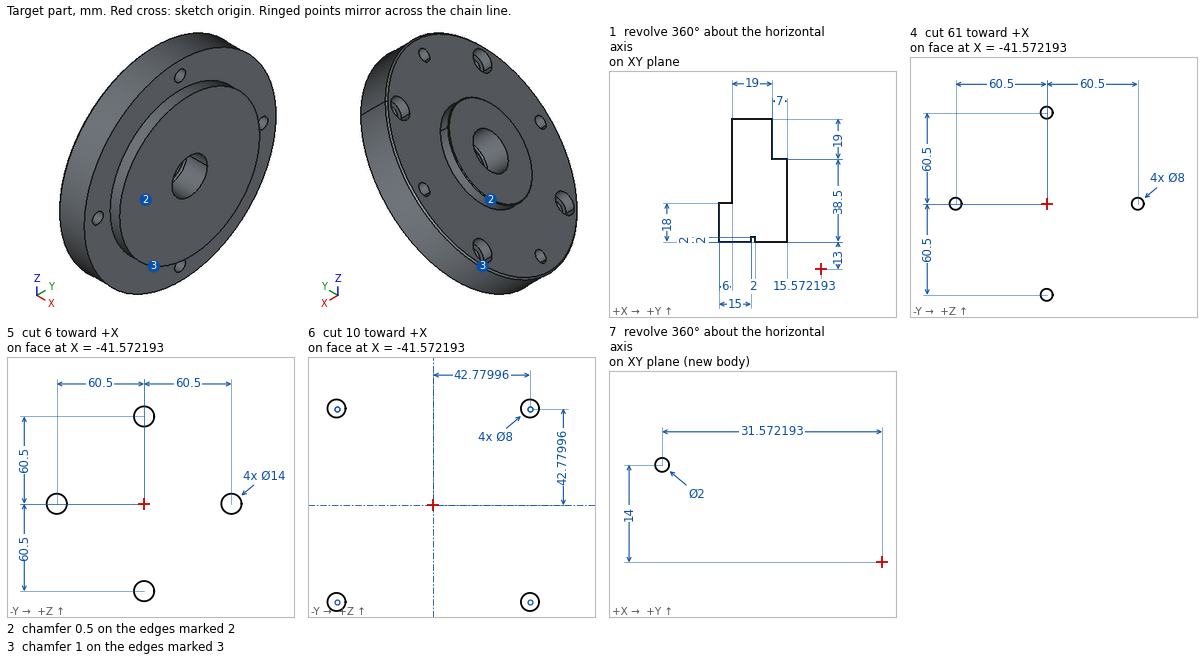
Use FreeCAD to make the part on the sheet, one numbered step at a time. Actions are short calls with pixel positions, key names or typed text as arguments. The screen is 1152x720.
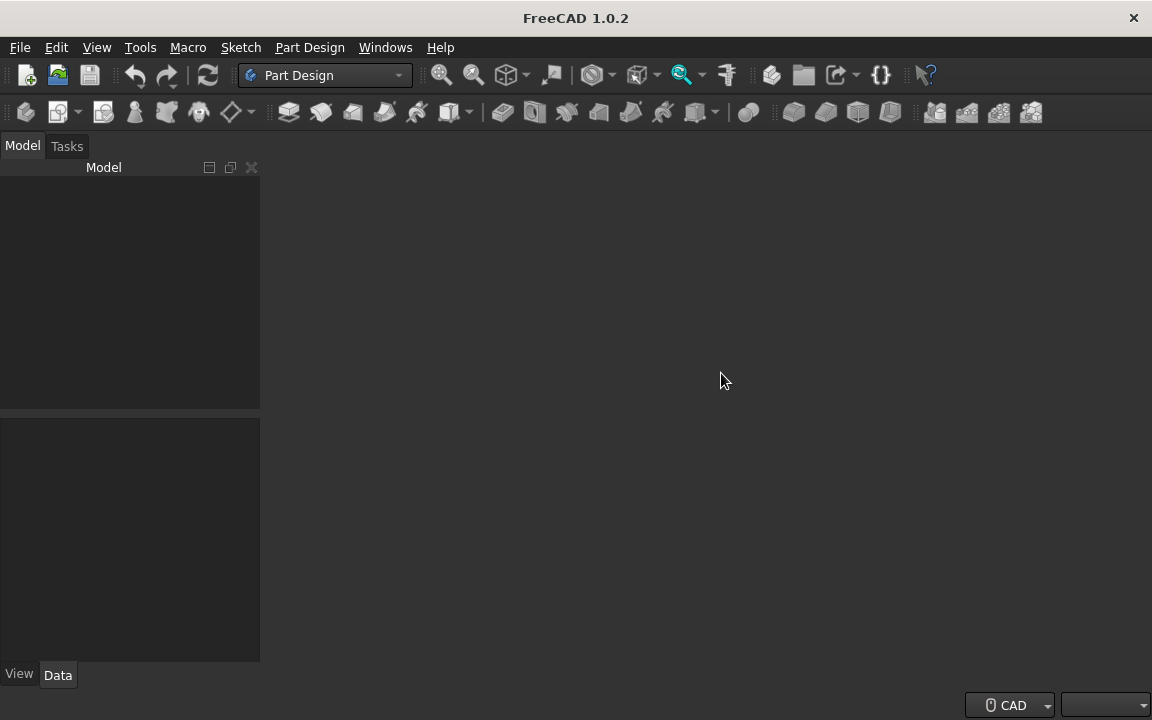
click(26, 76)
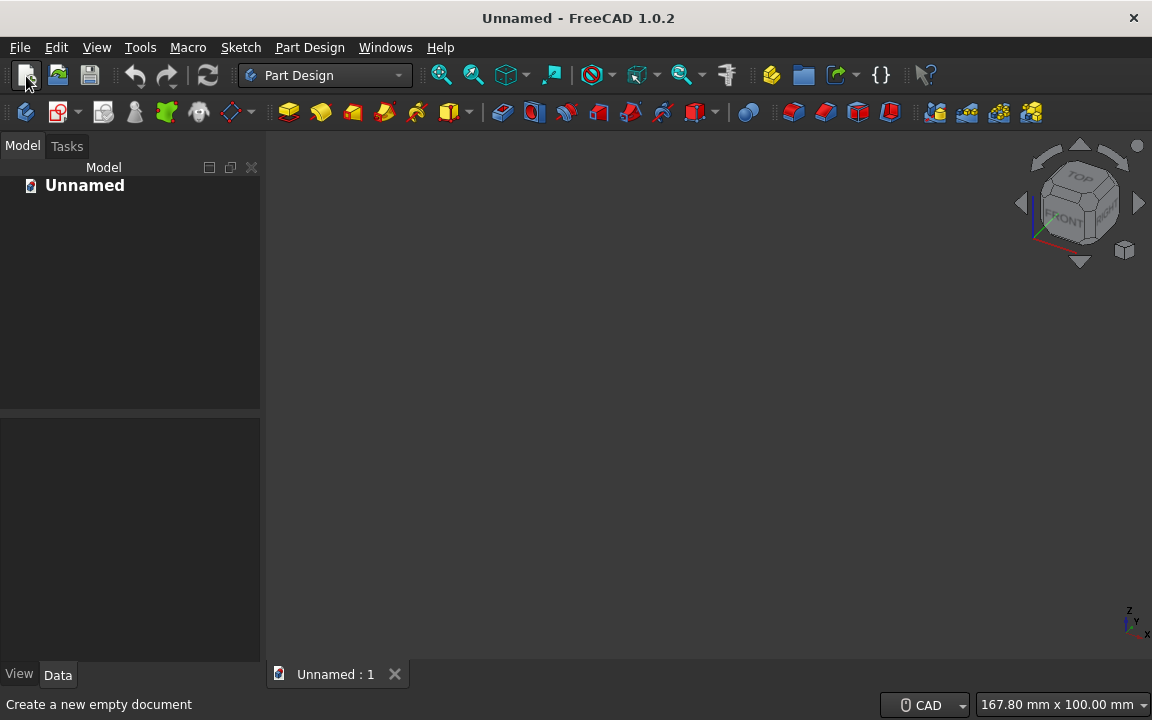
click(58, 112)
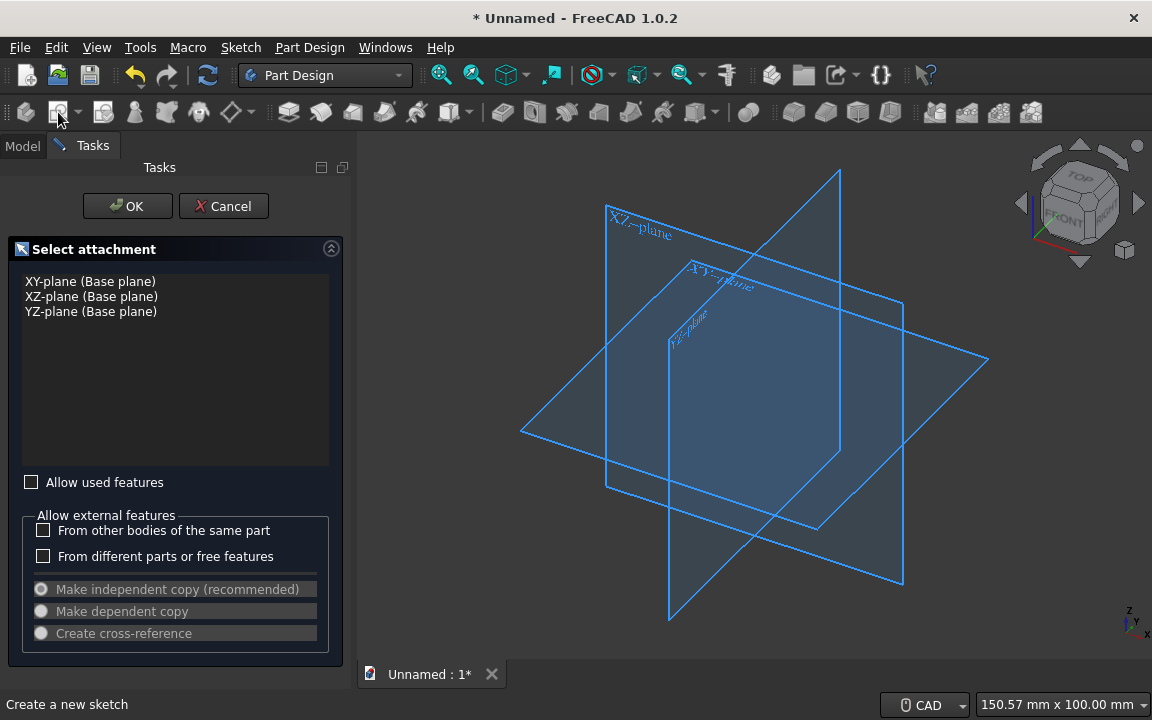
click(82, 282)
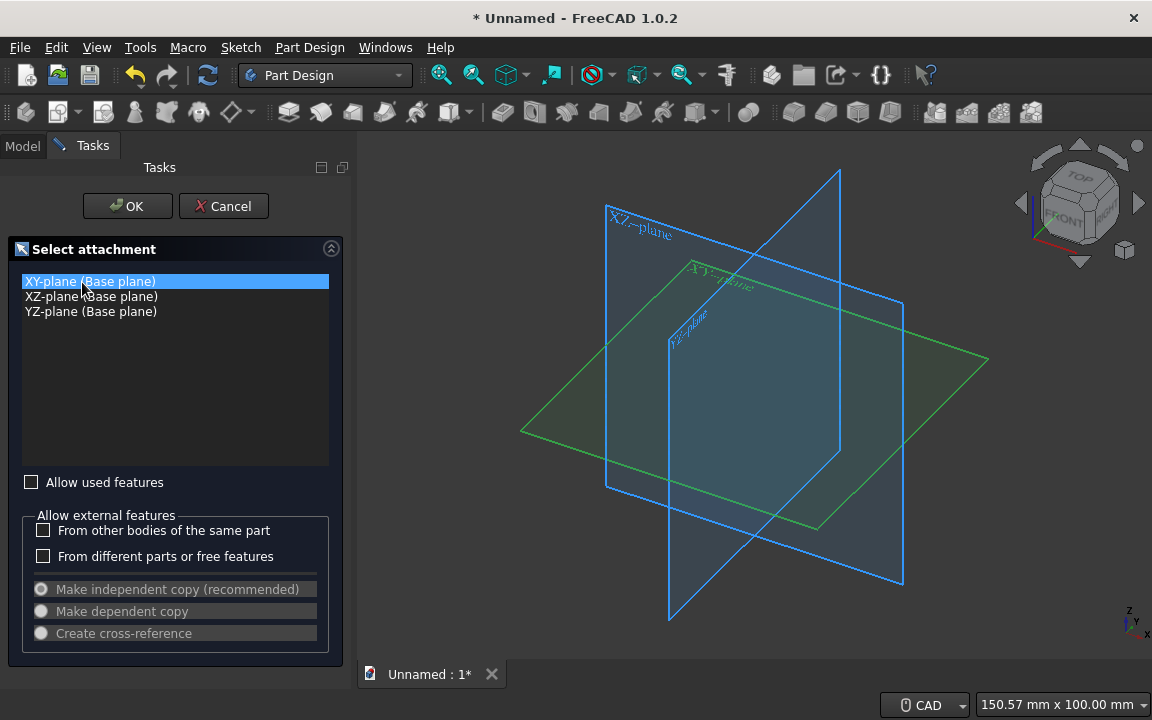
click(128, 206)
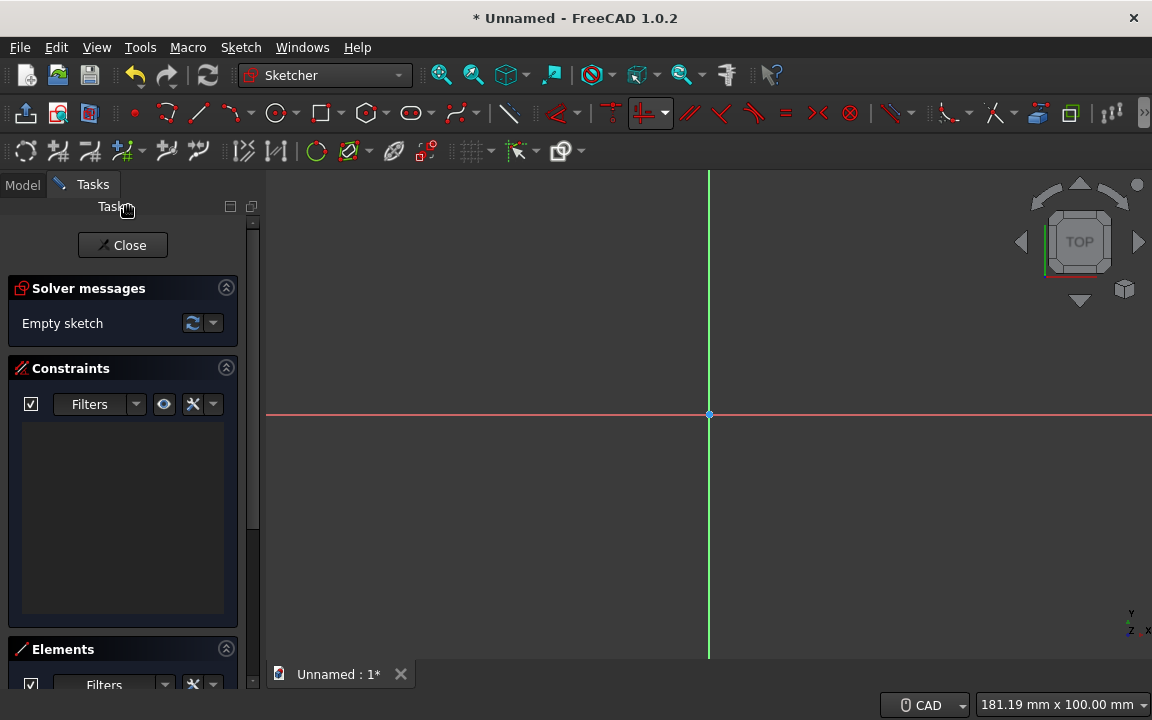
scroll(738, 631, down, 2)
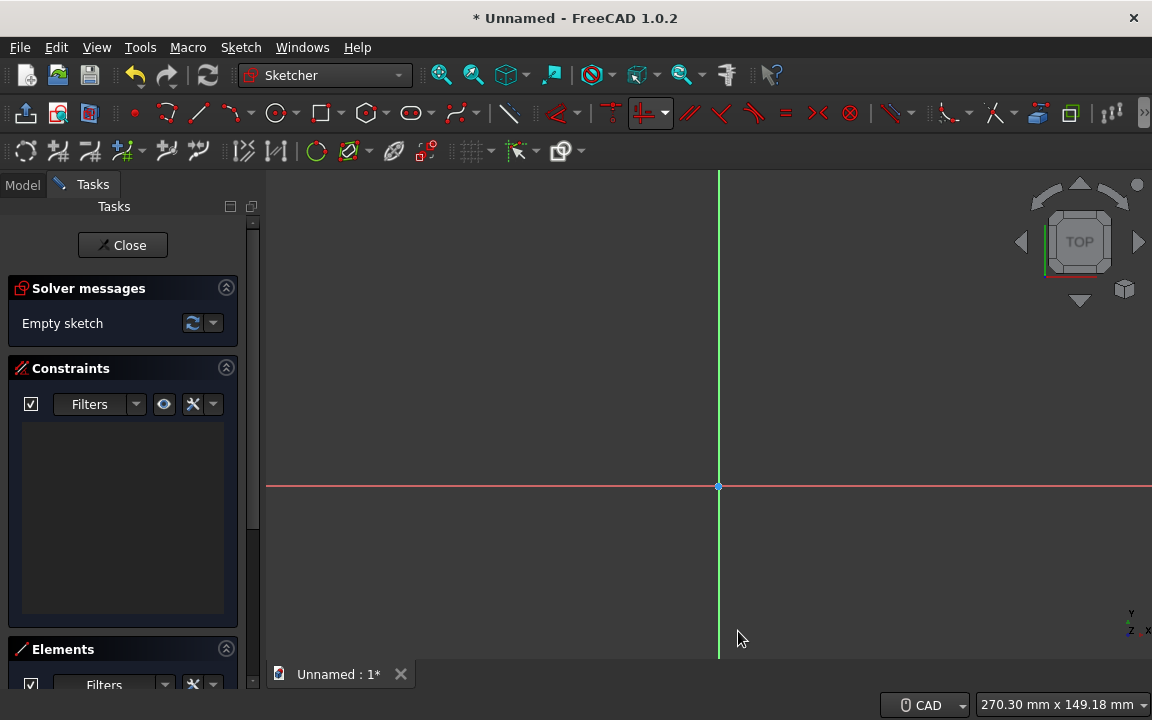
click(168, 114)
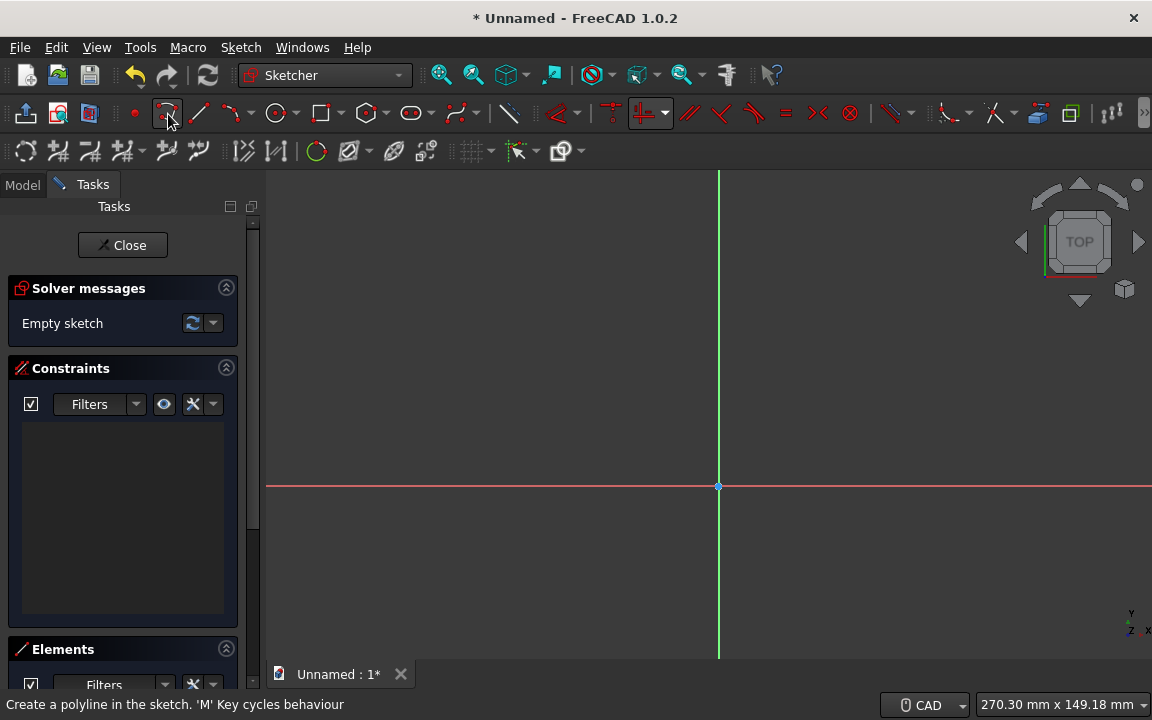
click(668, 444)
click(668, 317)
click(645, 317)
click(645, 255)
click(582, 255)
click(582, 385)
click(563, 385)
click(563, 444)
click(612, 444)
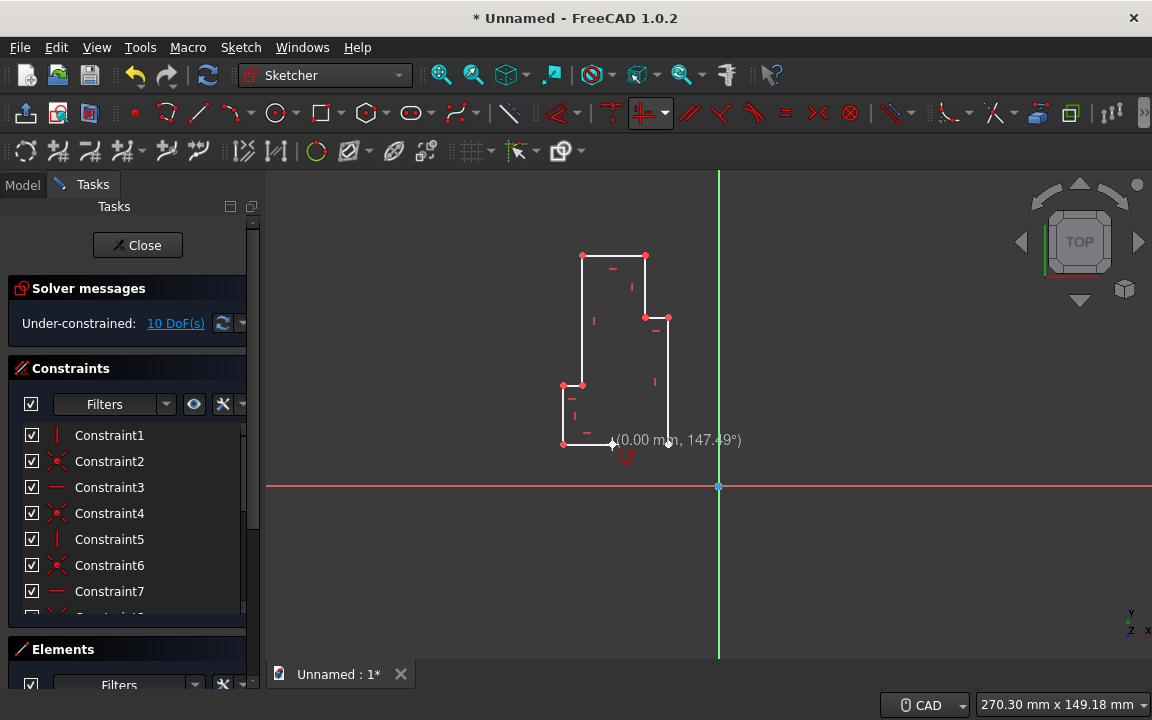
scroll(612, 437, up, 5)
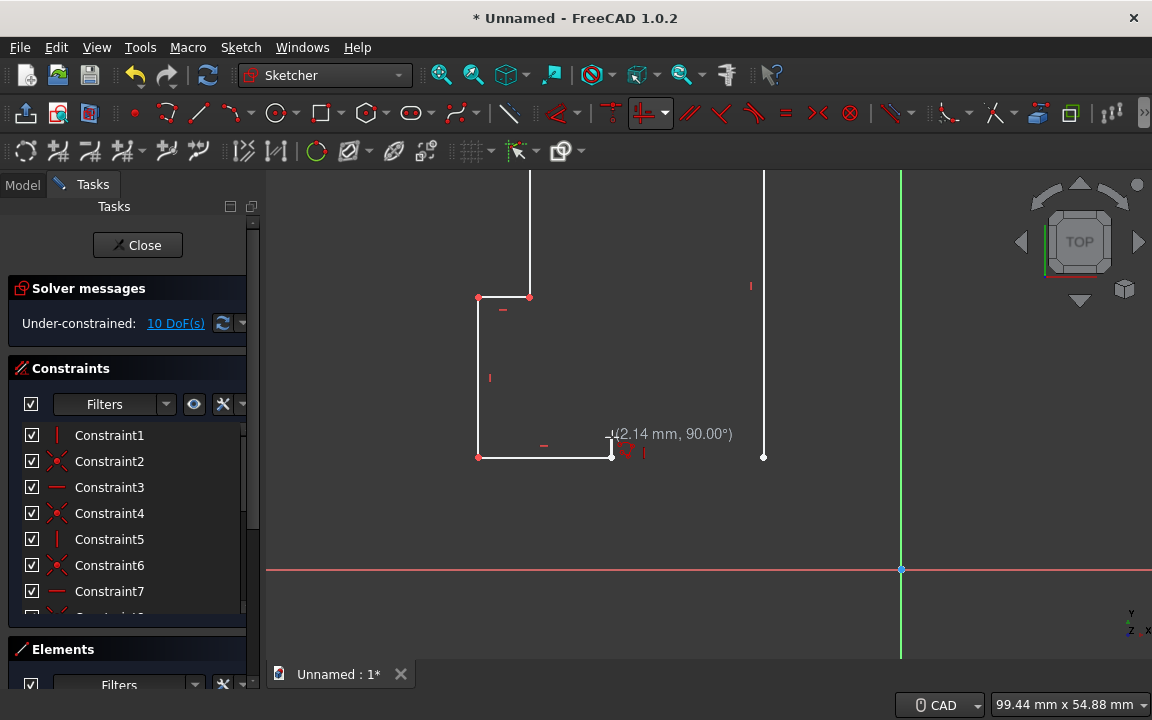
click(611, 436)
click(629, 436)
click(629, 454)
click(764, 458)
key(Escape)
key(Escape)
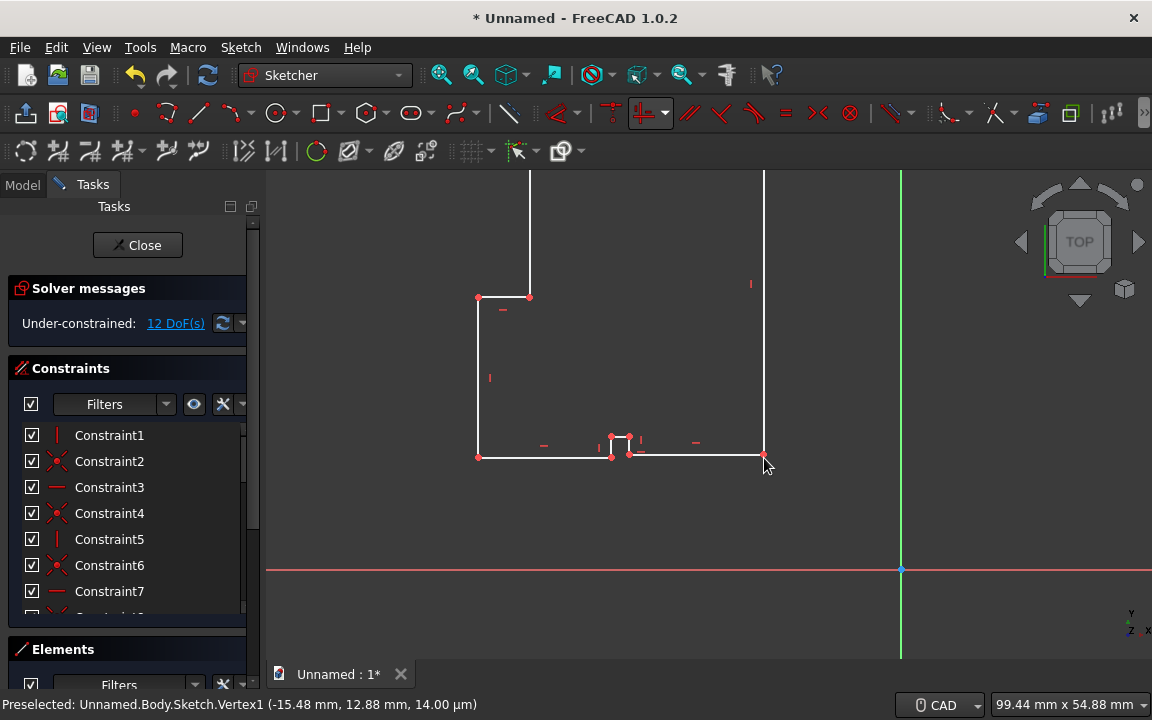
click(556, 114)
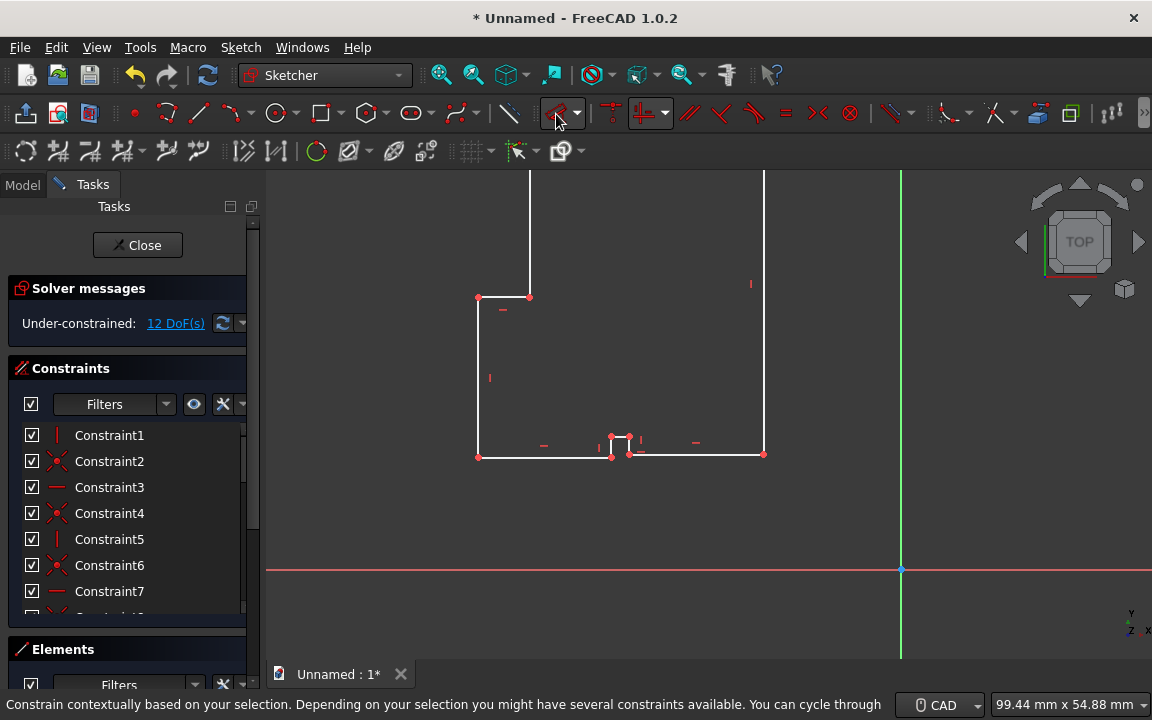
scroll(600, 544, down, 4)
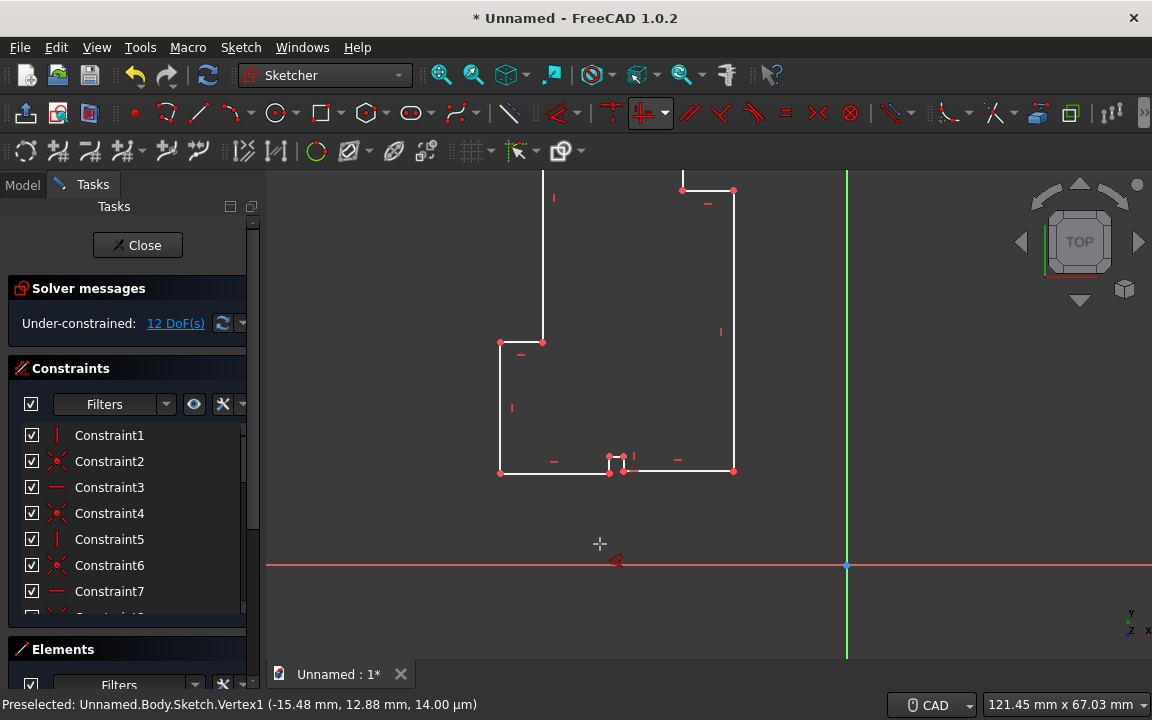
scroll(665, 351, up, 3)